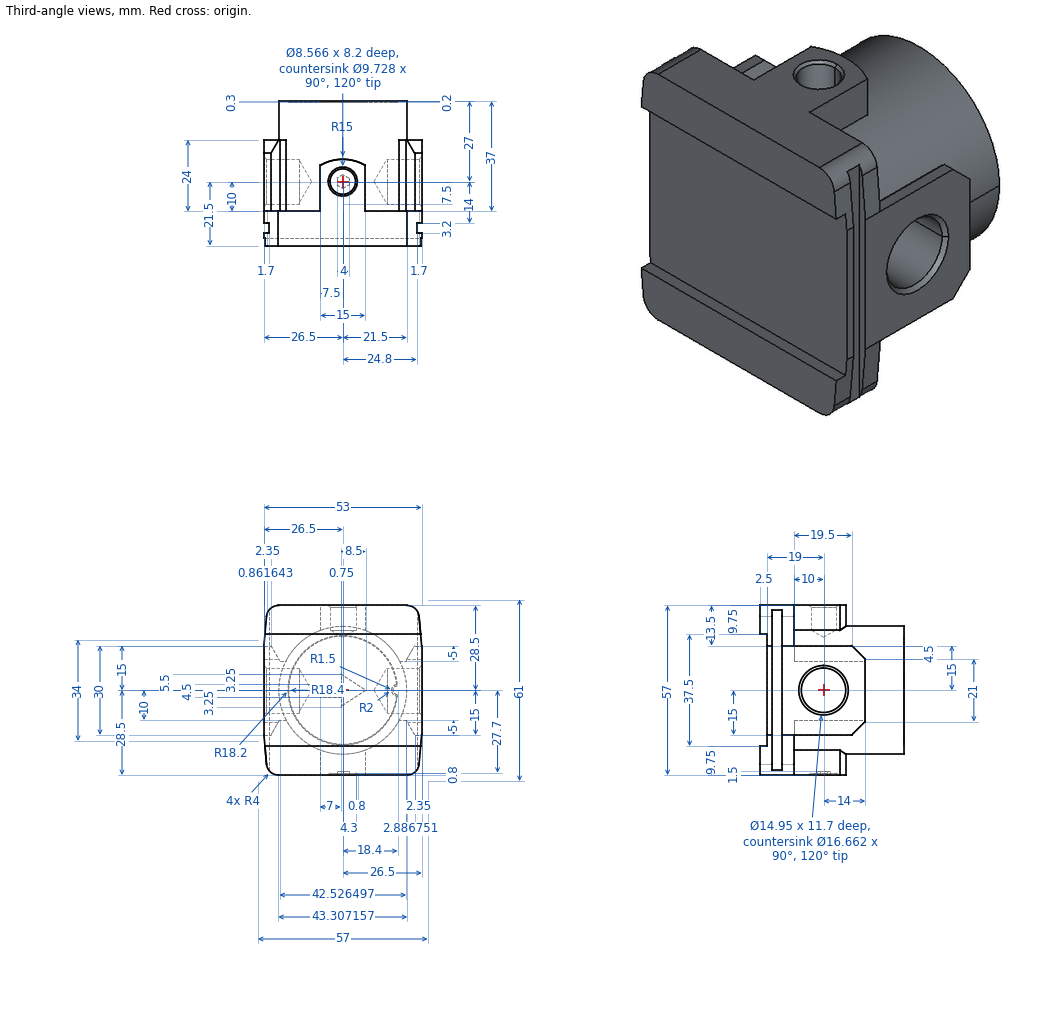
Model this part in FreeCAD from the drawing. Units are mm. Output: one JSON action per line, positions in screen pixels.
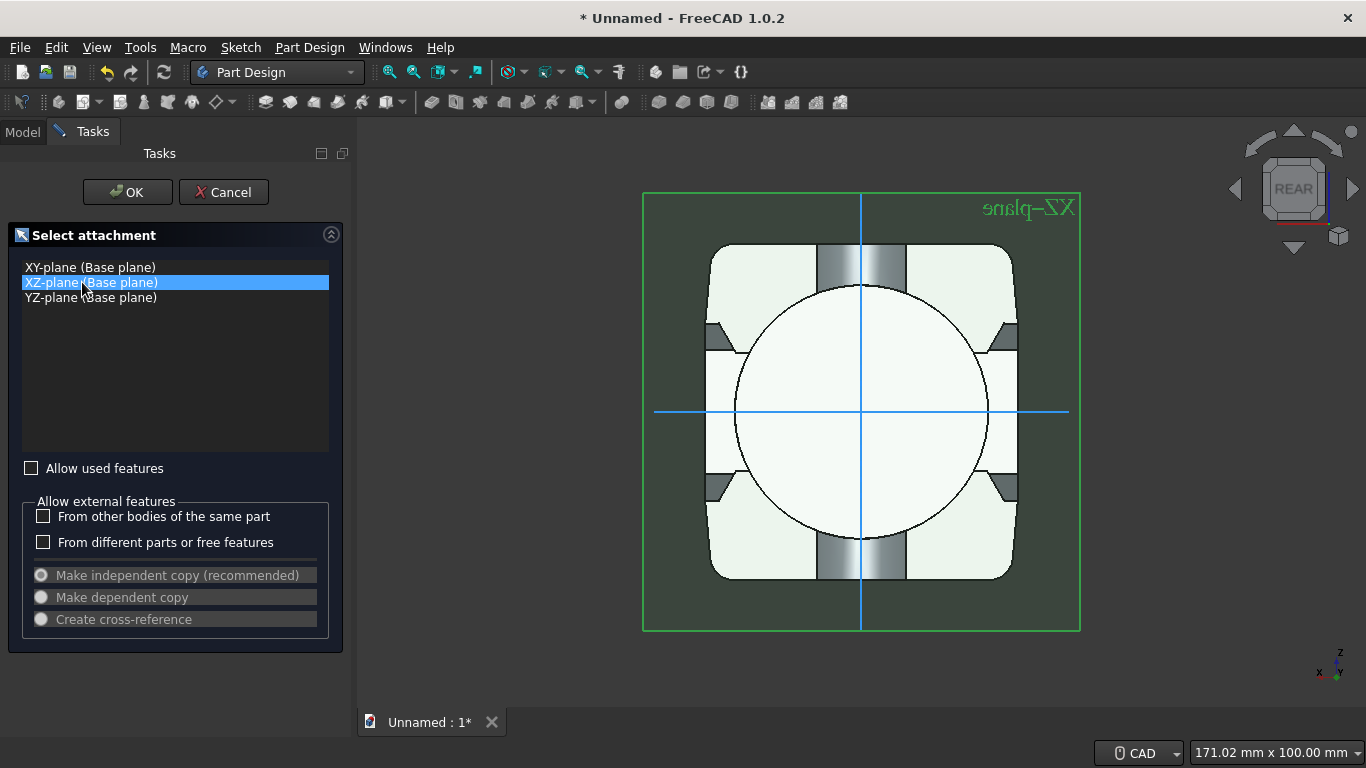
{"action": "left_click", "coordinate": [128, 192]}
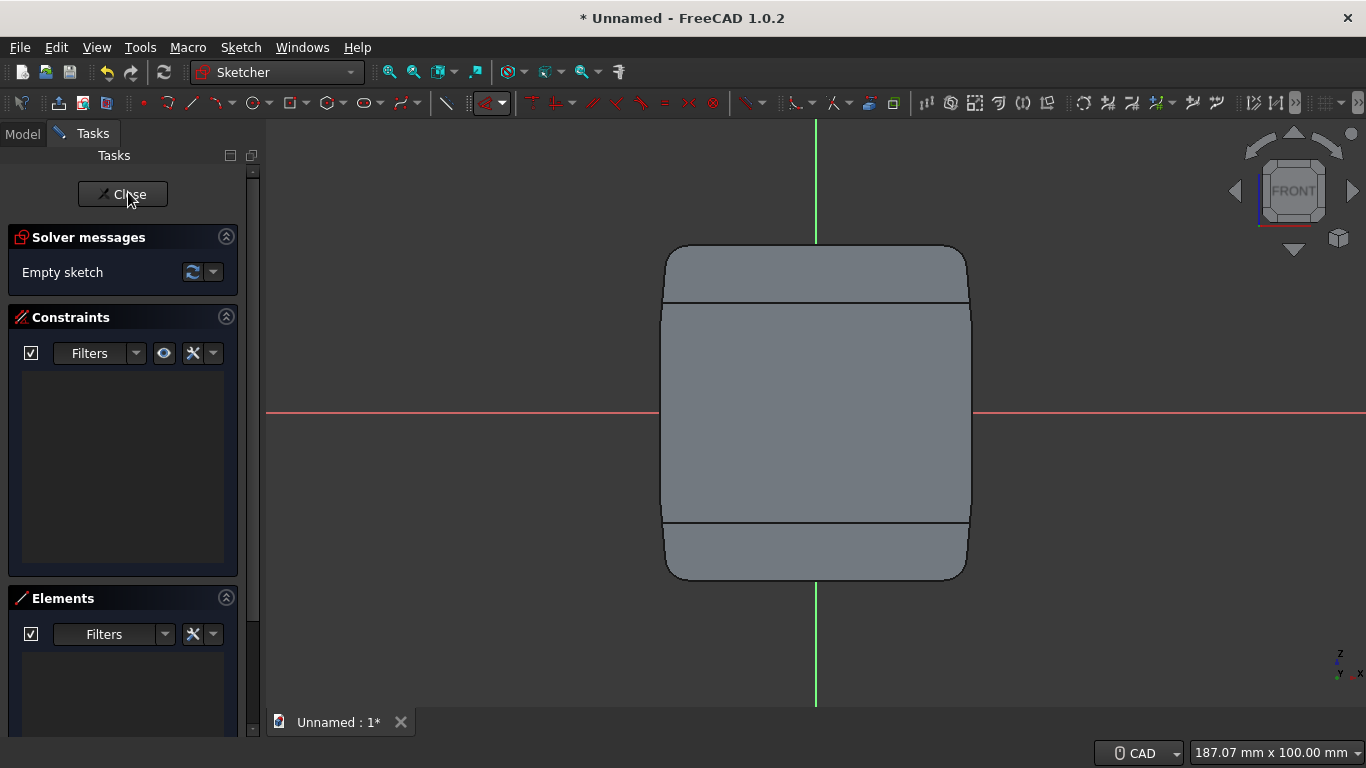
{"action": "left_click", "coordinate": [108, 104]}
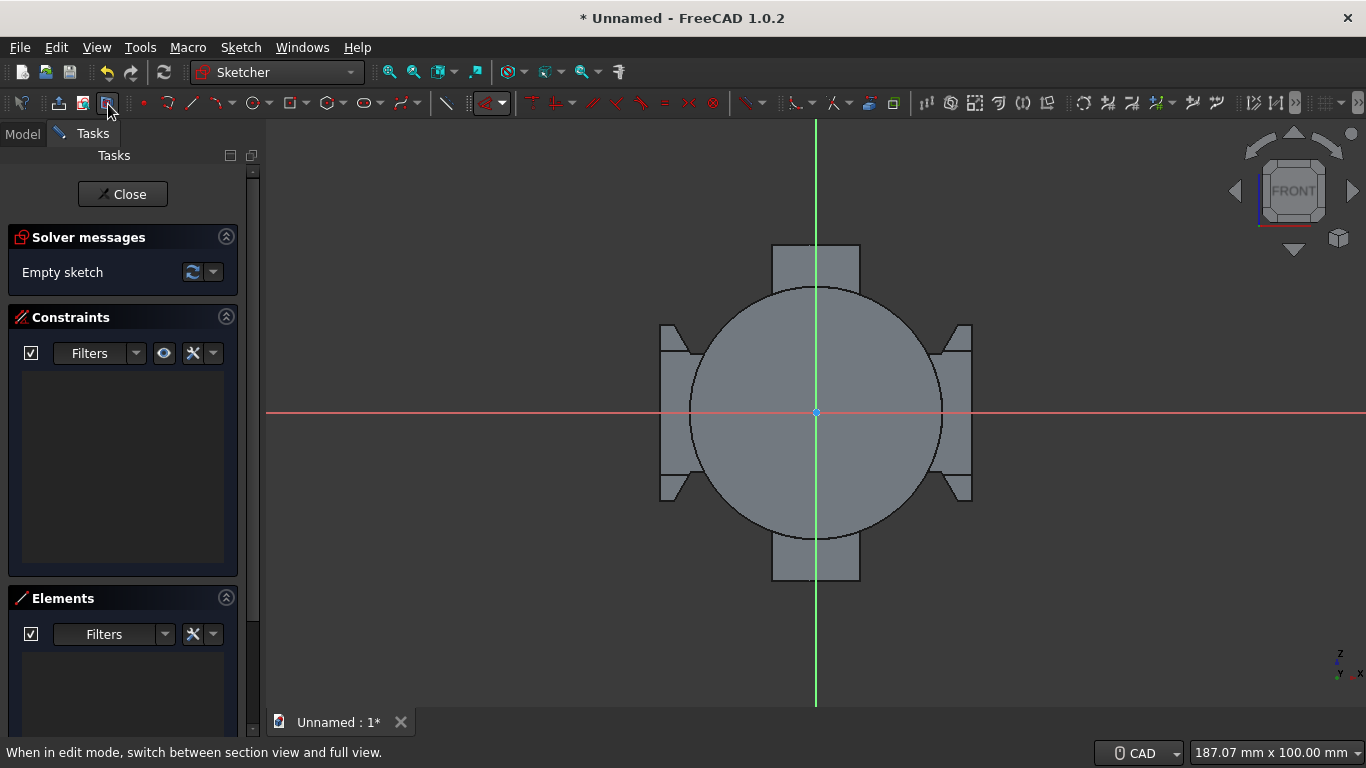
{"action": "scroll", "coordinate": [849, 587], "scroll_direction": "up", "scroll_amount": 15}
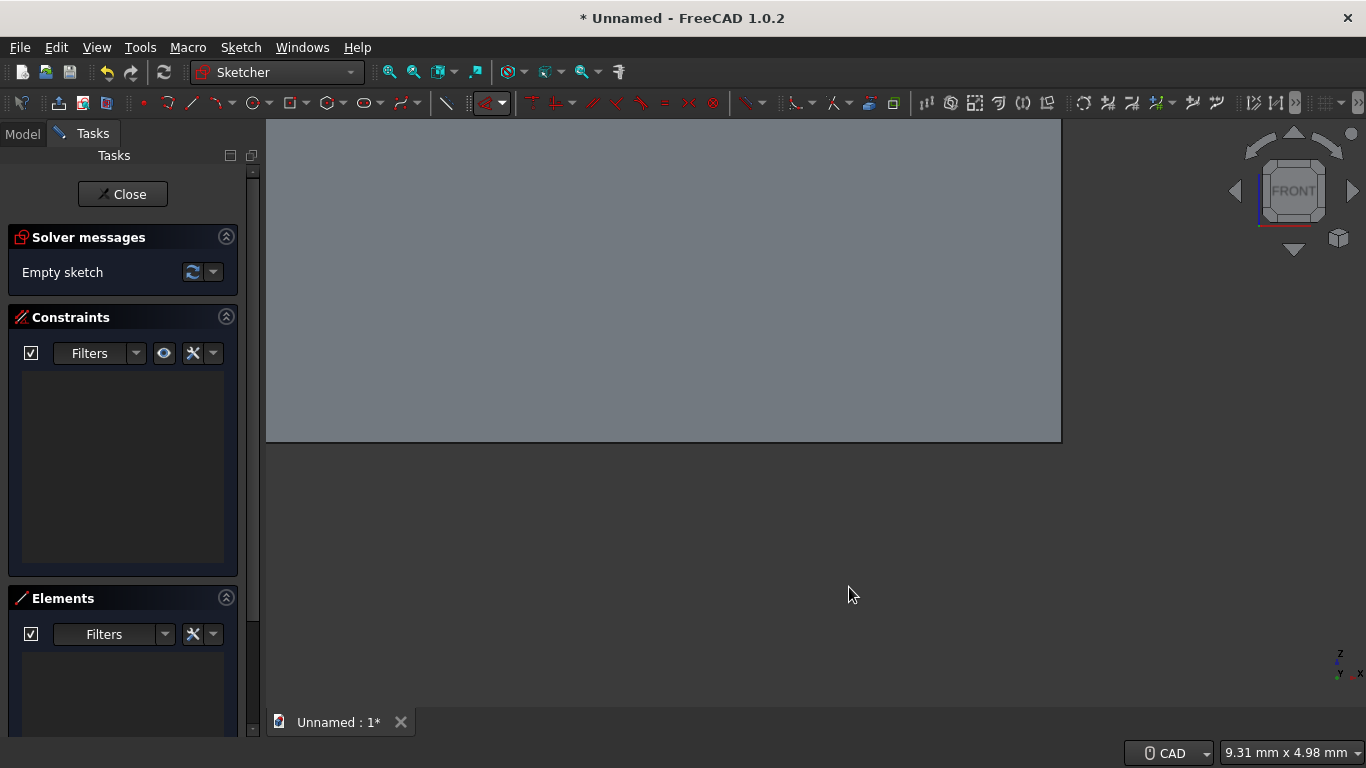
{"action": "scroll", "coordinate": [726, 390], "scroll_direction": "up", "scroll_amount": 7}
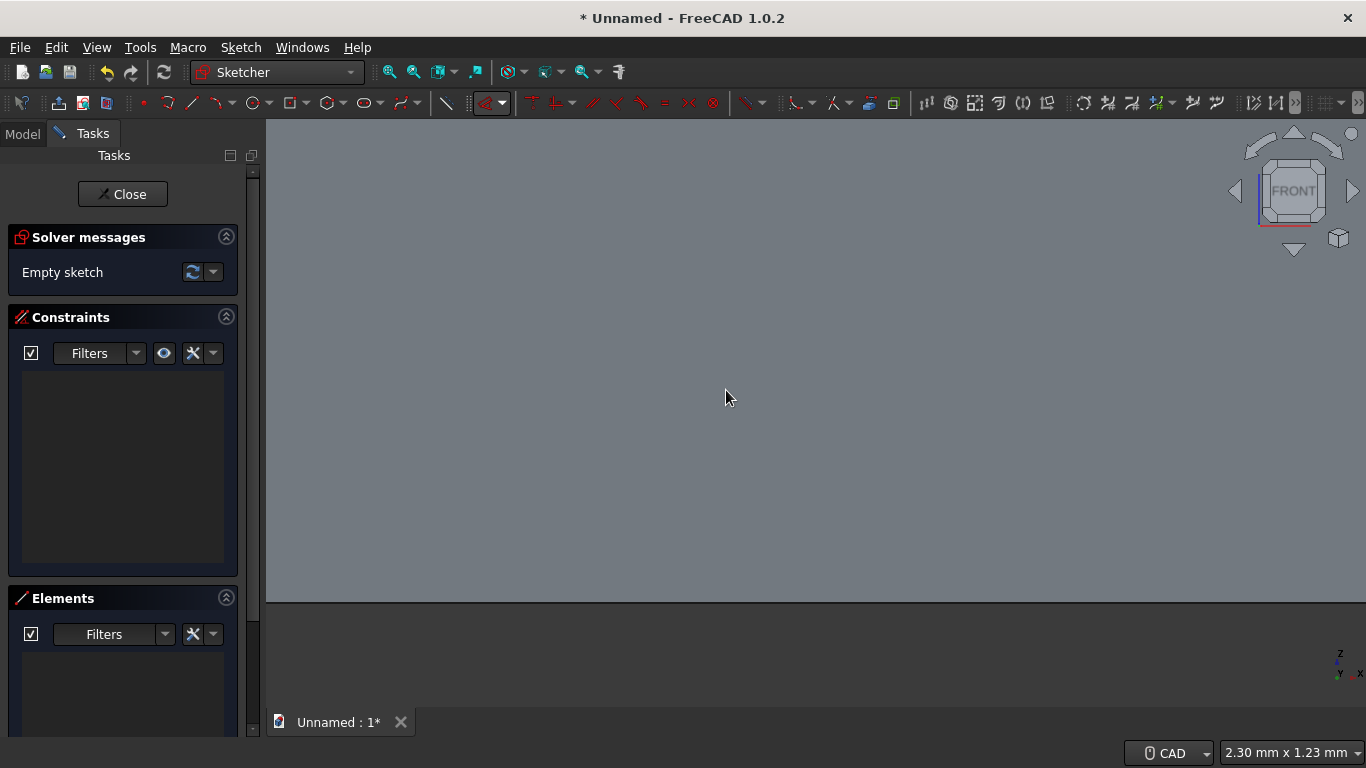
{"action": "left_click", "coordinate": [168, 104]}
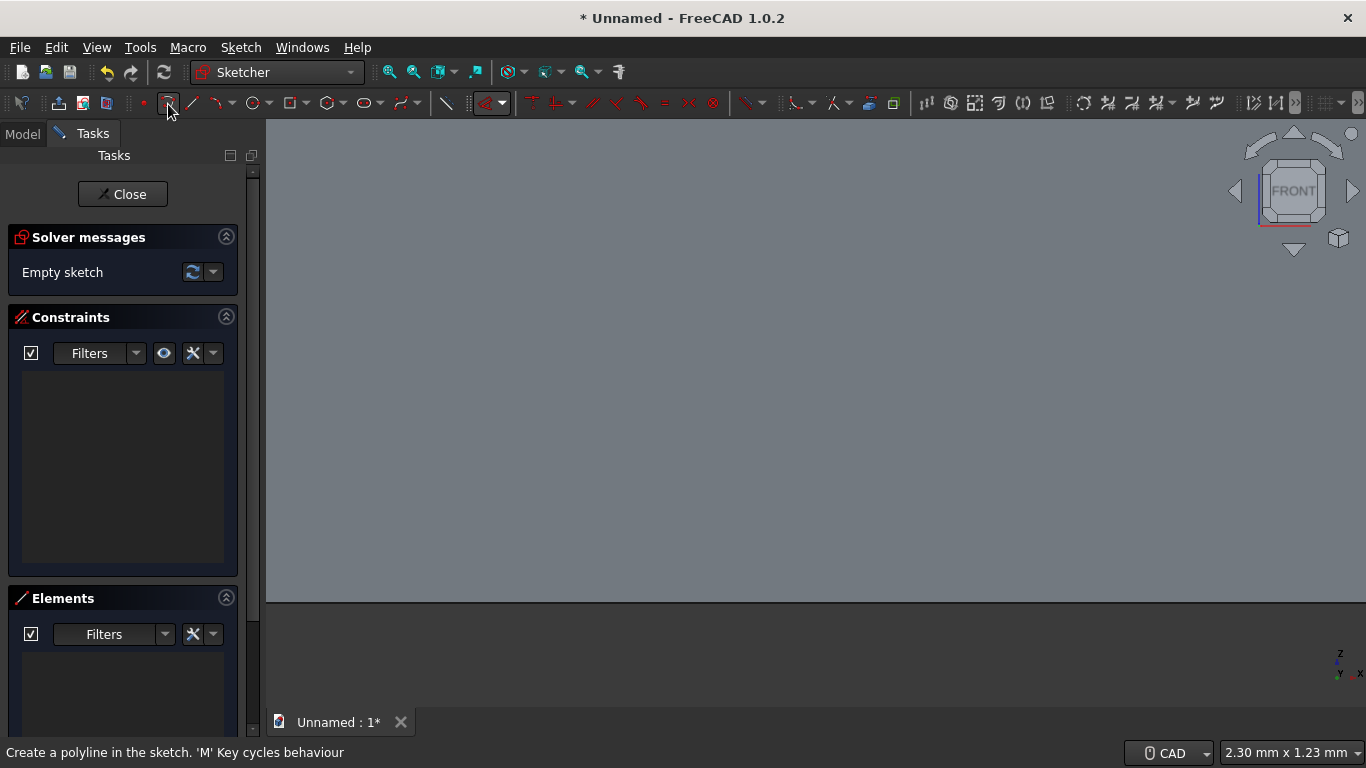
{"action": "left_click", "coordinate": [554, 220]}
{"action": "left_click", "coordinate": [937, 603]}
{"action": "left_click", "coordinate": [554, 603]}
{"action": "left_click", "coordinate": [554, 221]}
{"action": "key", "text": "Escape"}
{"action": "key", "text": "Escape"}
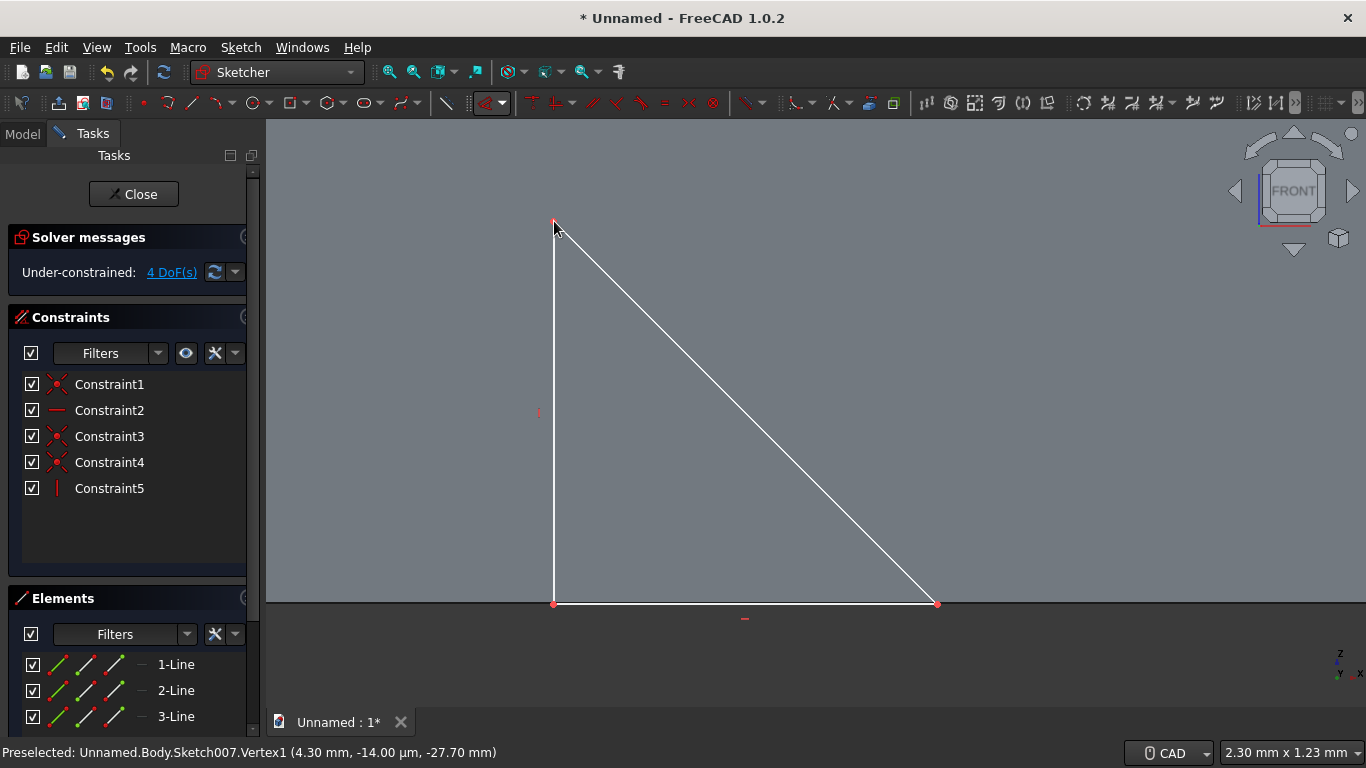
{"action": "left_click", "coordinate": [822, 604]}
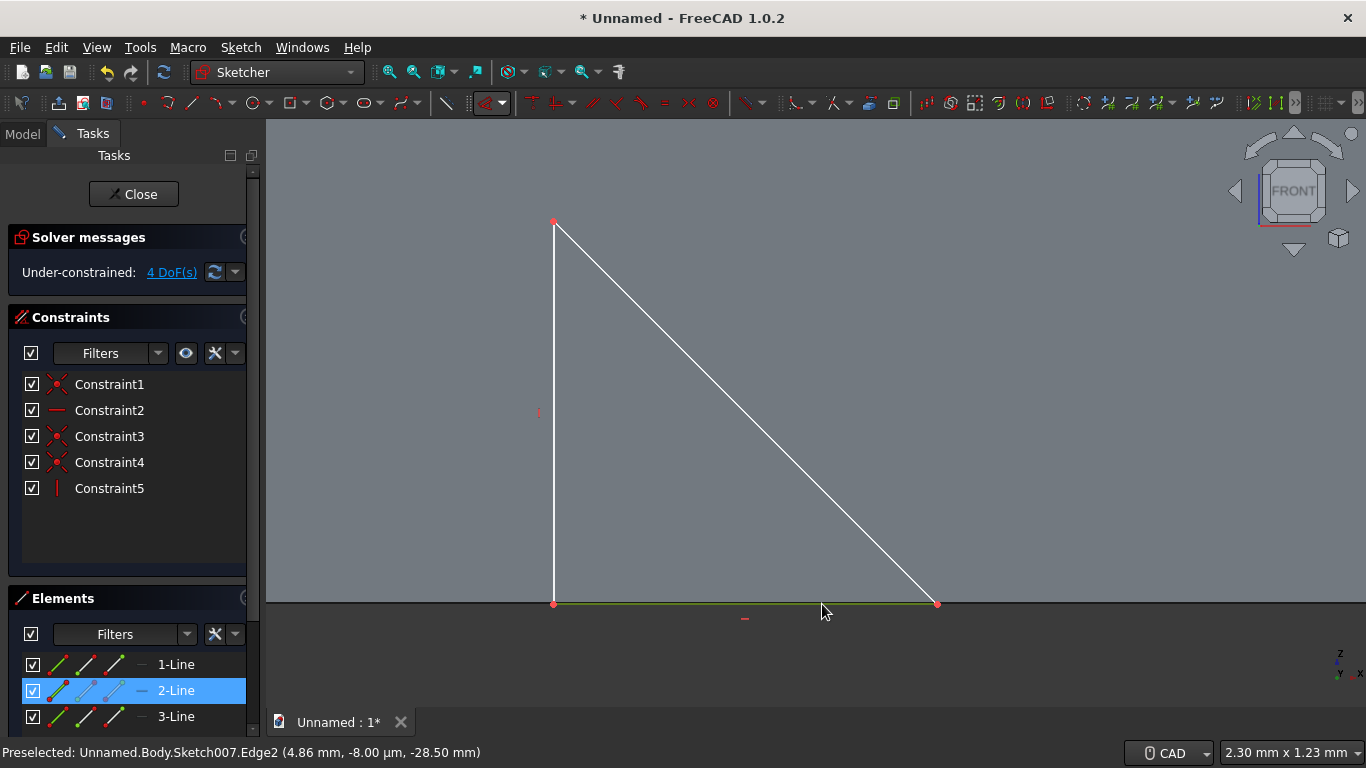
{"action": "left_click", "coordinate": [504, 104]}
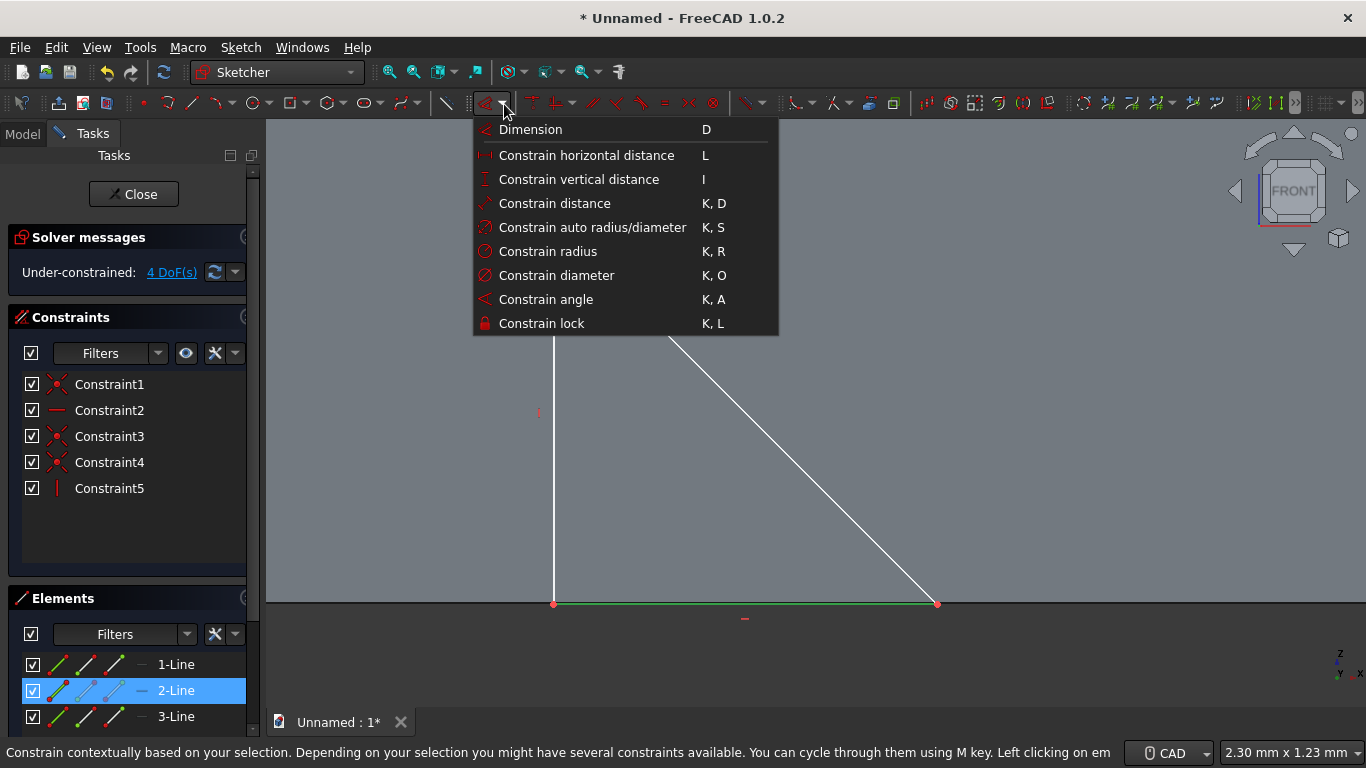
{"action": "left_click", "coordinate": [626, 155]}